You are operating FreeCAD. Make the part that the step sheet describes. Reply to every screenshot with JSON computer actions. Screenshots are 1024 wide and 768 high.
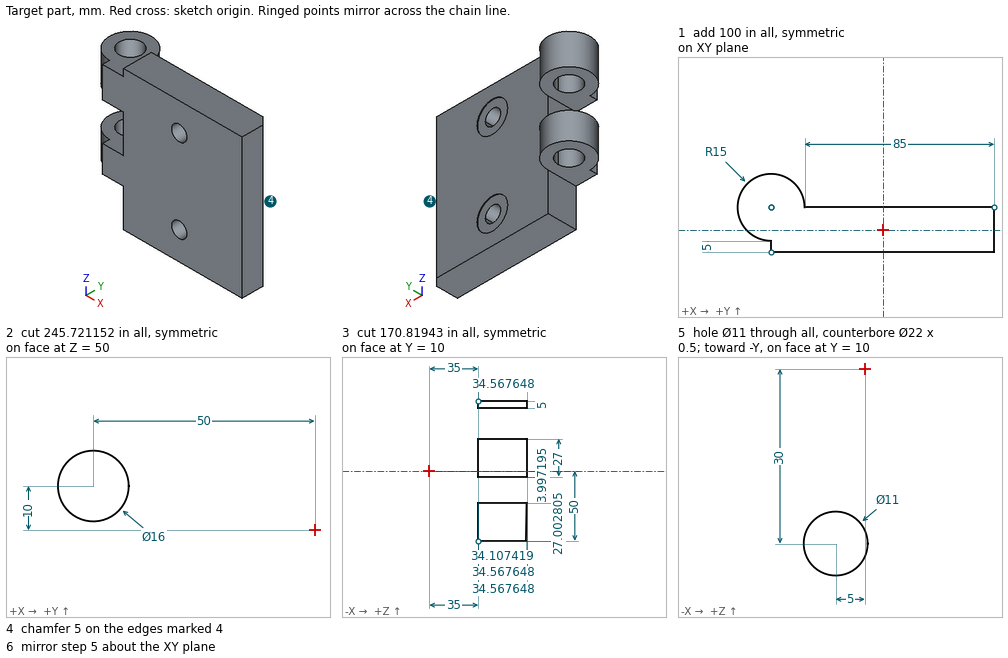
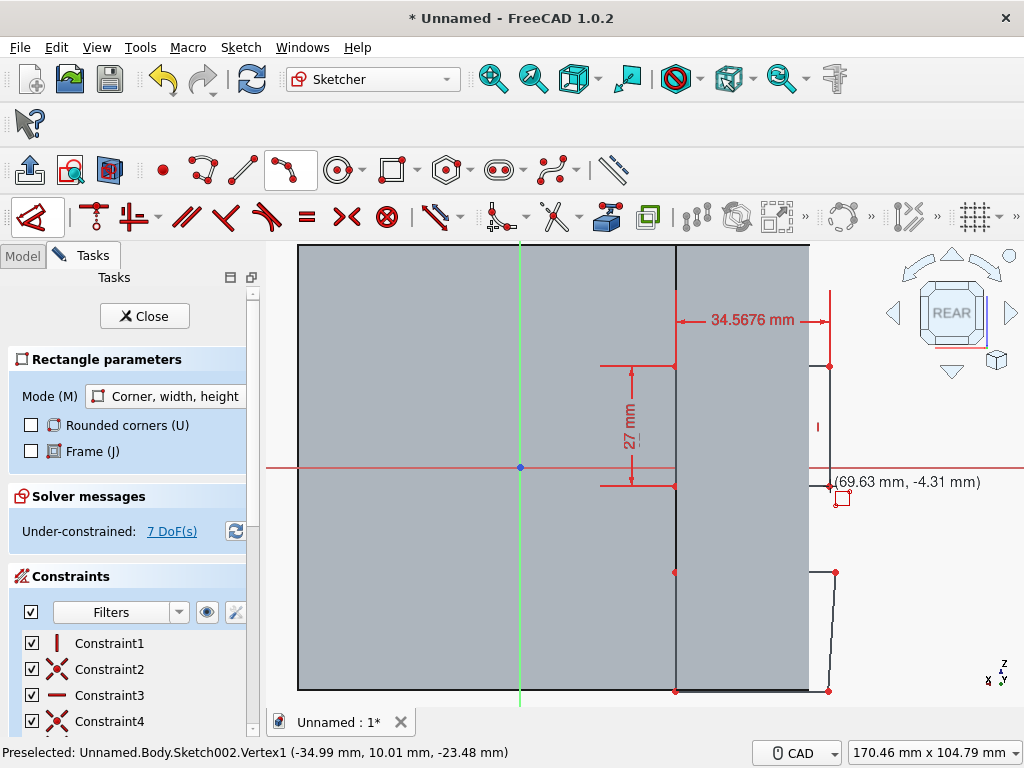
{"action": "scroll", "coordinate": [376, 487], "scroll_direction": "down", "scroll_amount": 2}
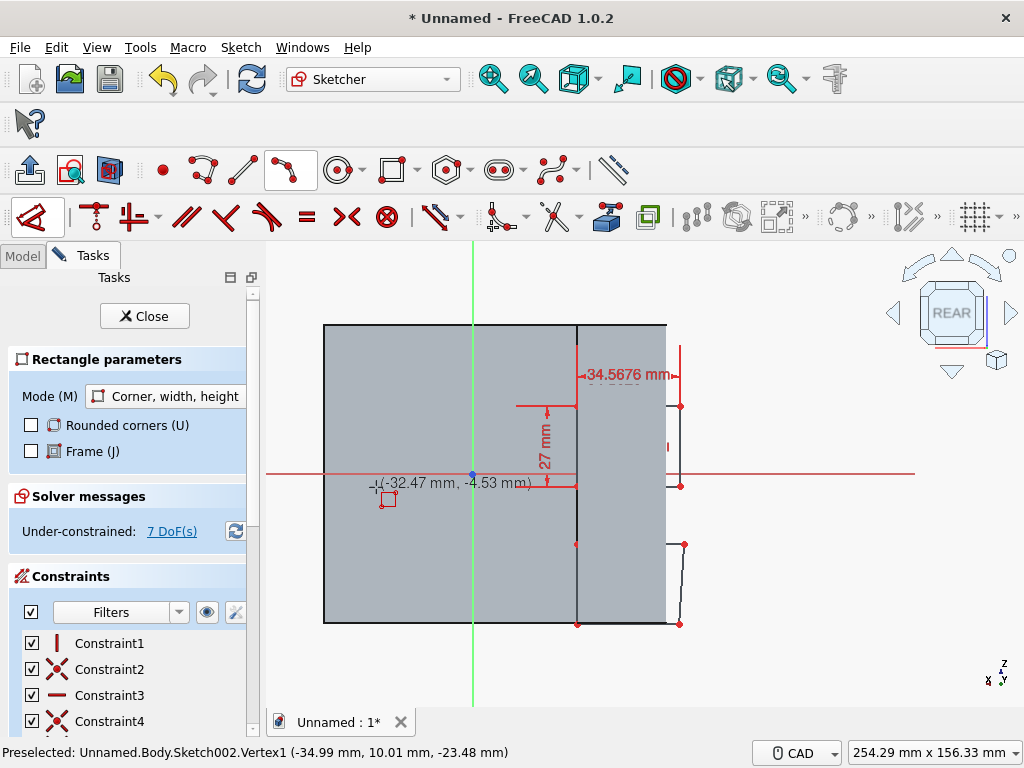
{"action": "left_click", "coordinate": [577, 325]}
{"action": "mouse_move", "coordinate": [680, 340]}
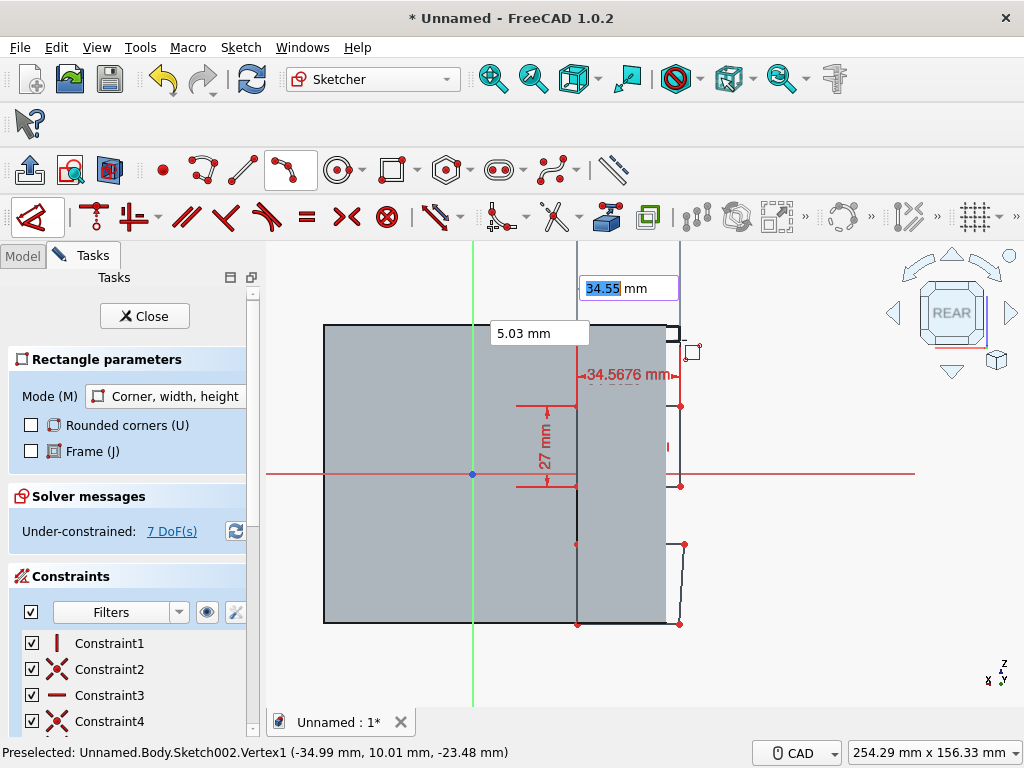
{"action": "type", "text": "34.567648"}
{"action": "key", "text": "Tab"}
{"action": "type", "text": "5"}
{"action": "key", "text": "Return"}
{"action": "key", "text": "Escape"}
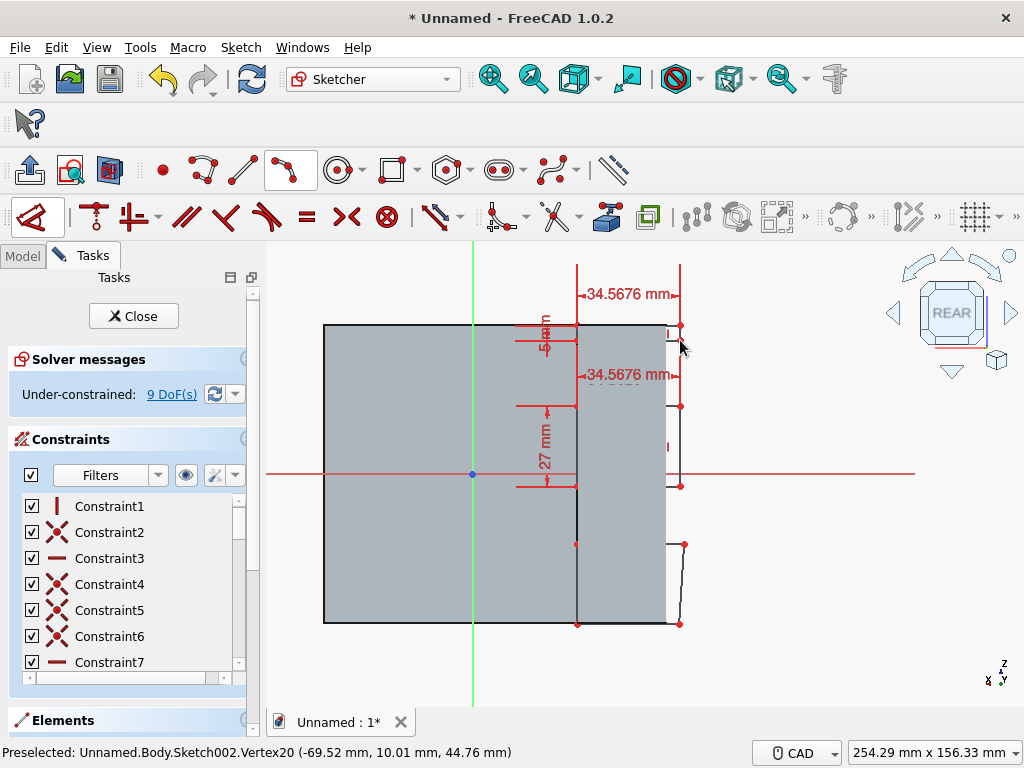
{"action": "left_click", "coordinate": [577, 624]}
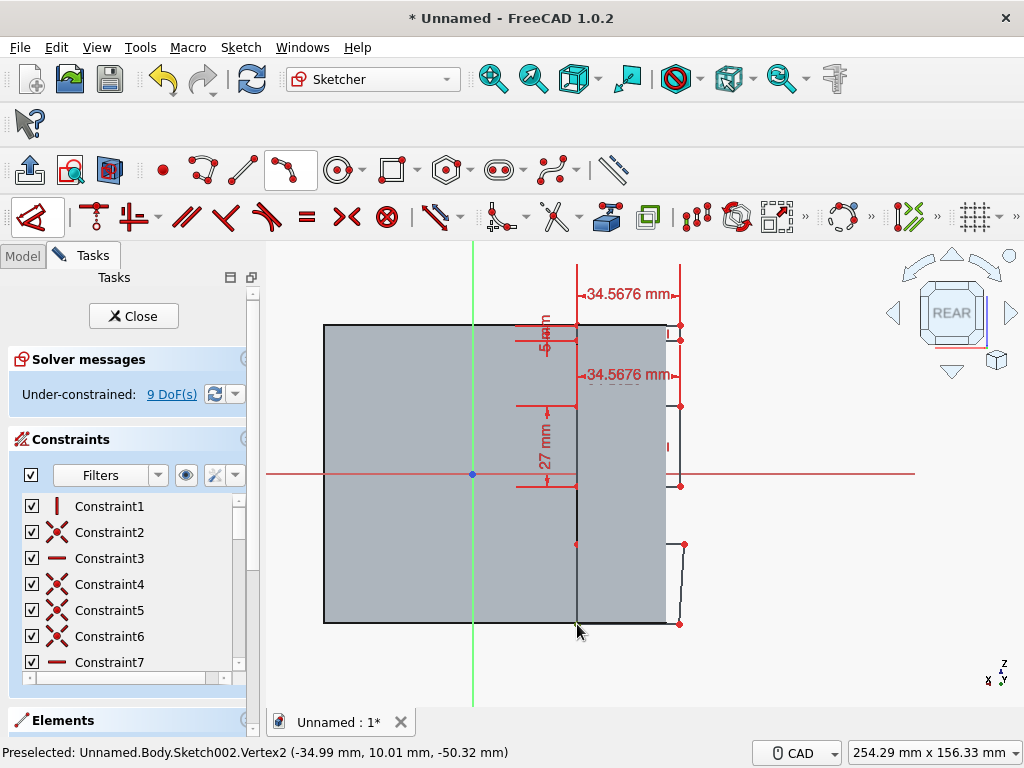
{"action": "left_click", "coordinate": [577, 326]}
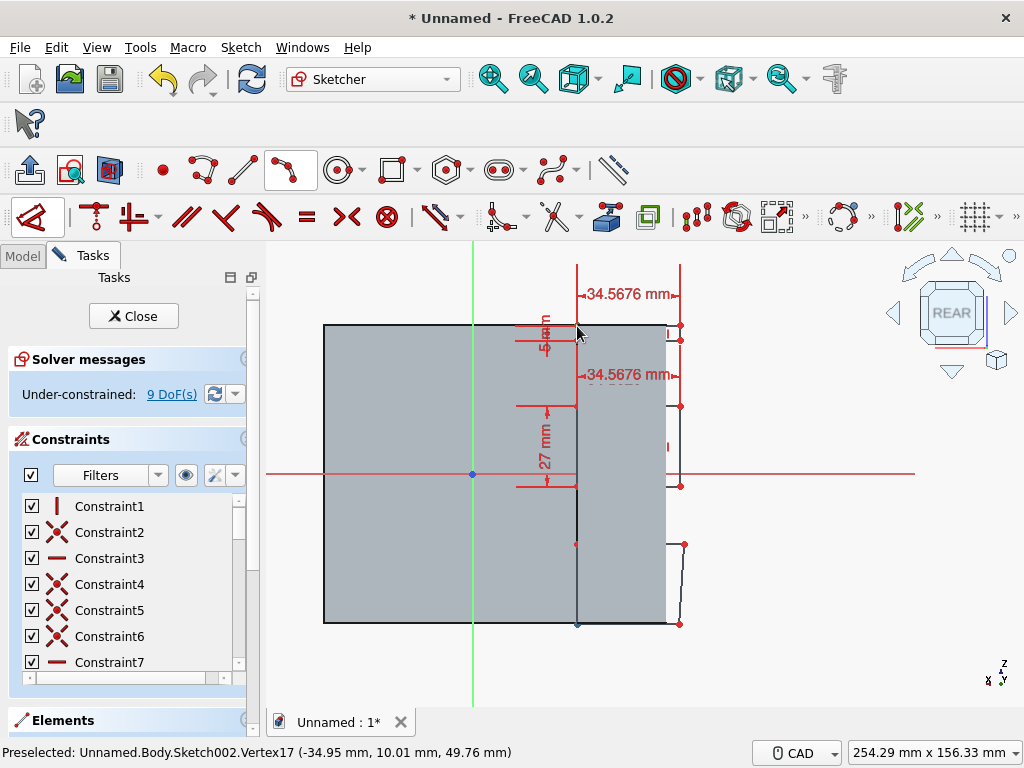
{"action": "left_click", "coordinate": [334, 474]}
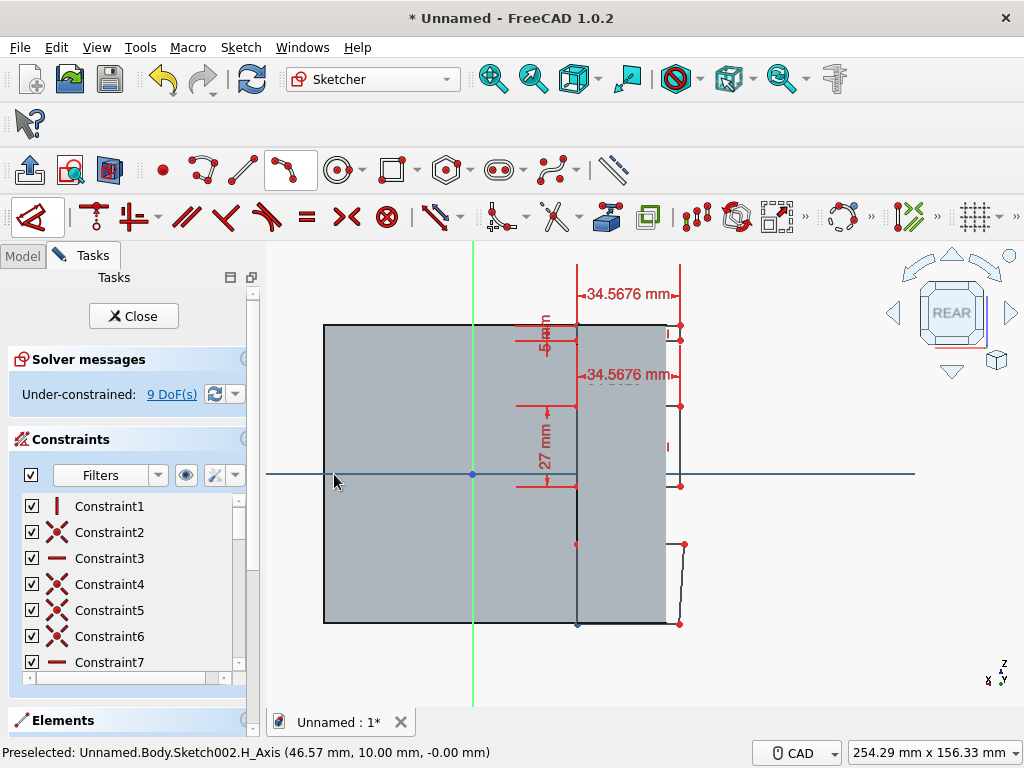
{"action": "left_click", "coordinate": [348, 218]}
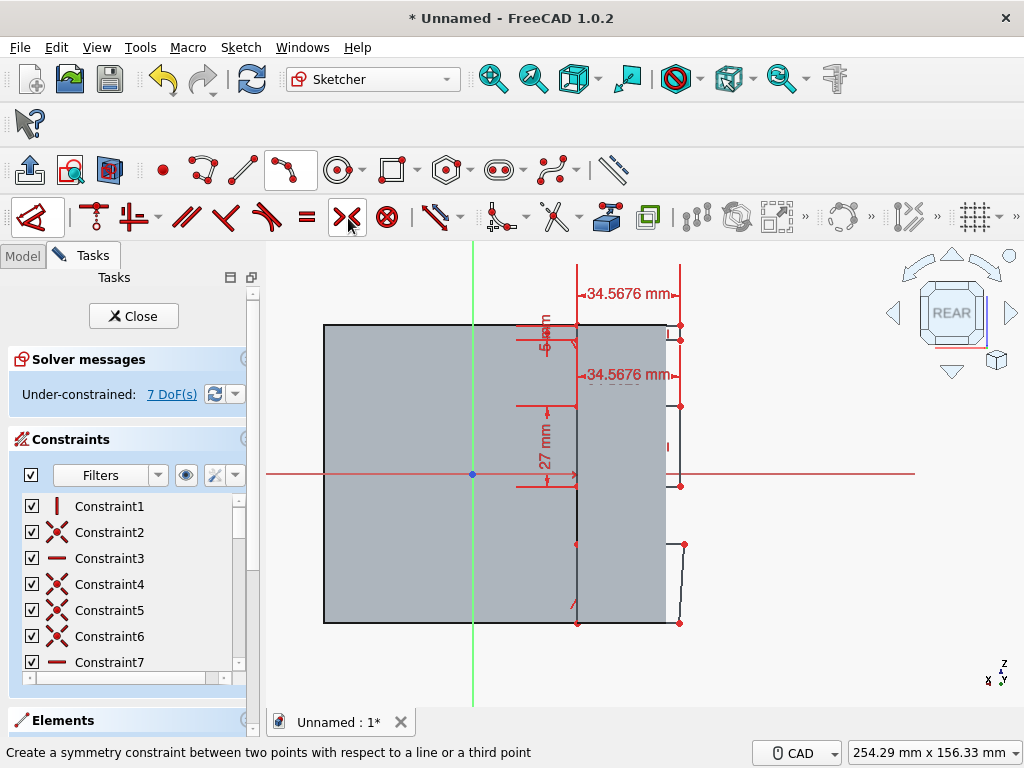
{"action": "left_click", "coordinate": [577, 544]}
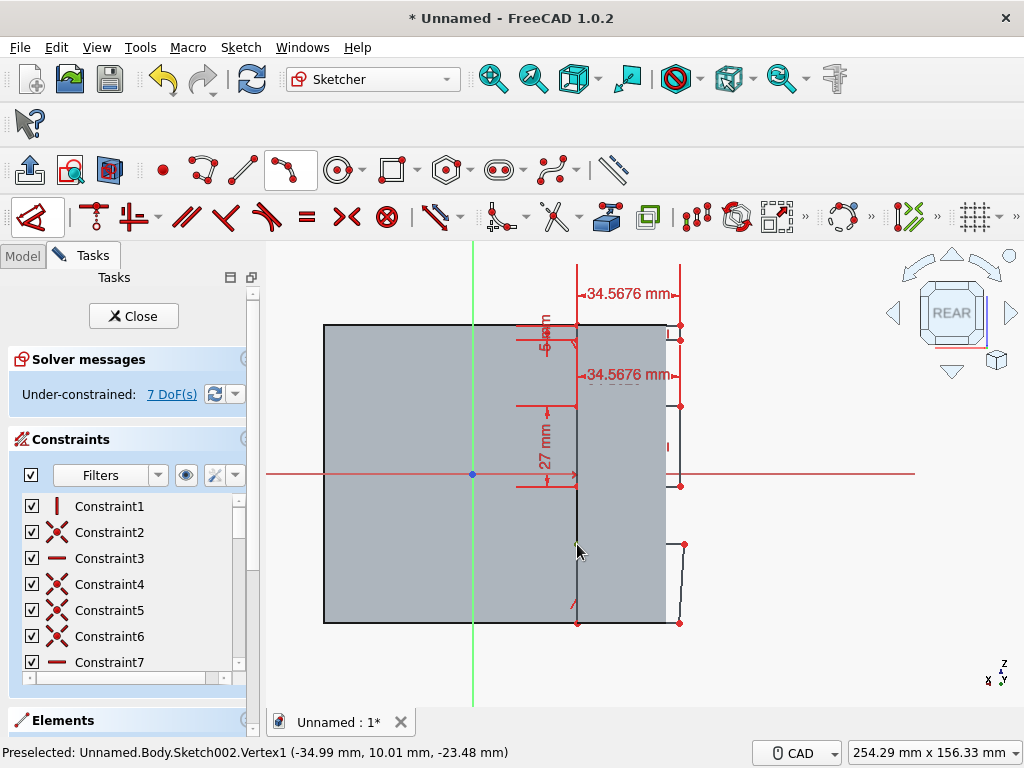
{"action": "left_click", "coordinate": [58, 218]}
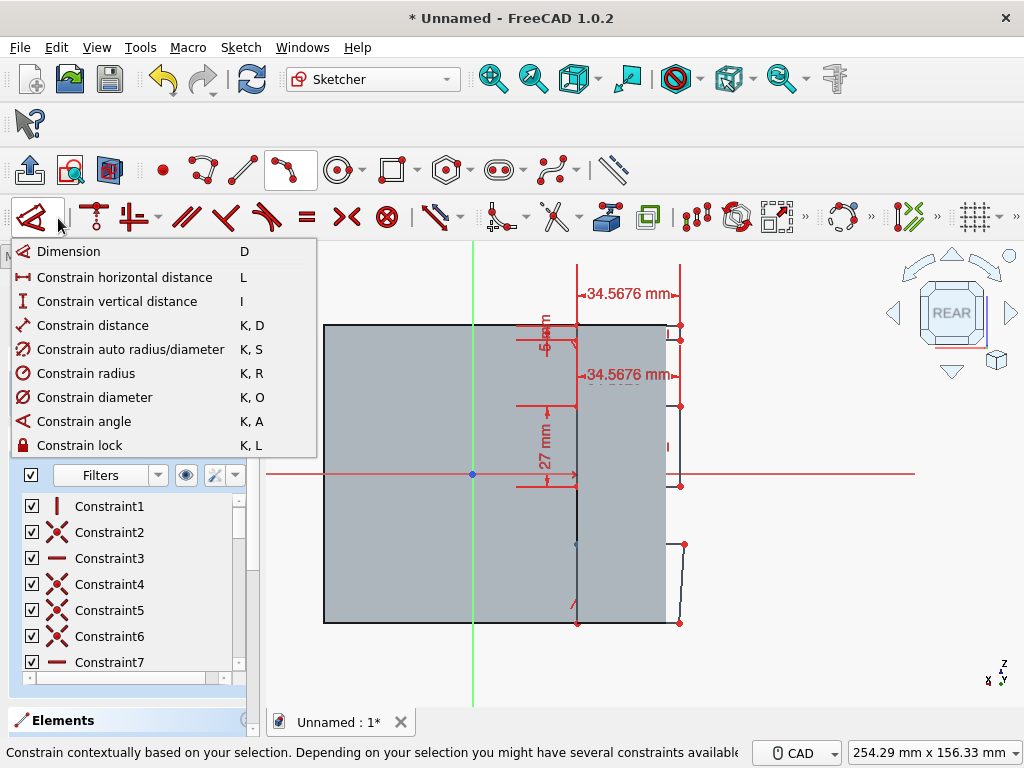
{"action": "left_click", "coordinate": [164, 277]}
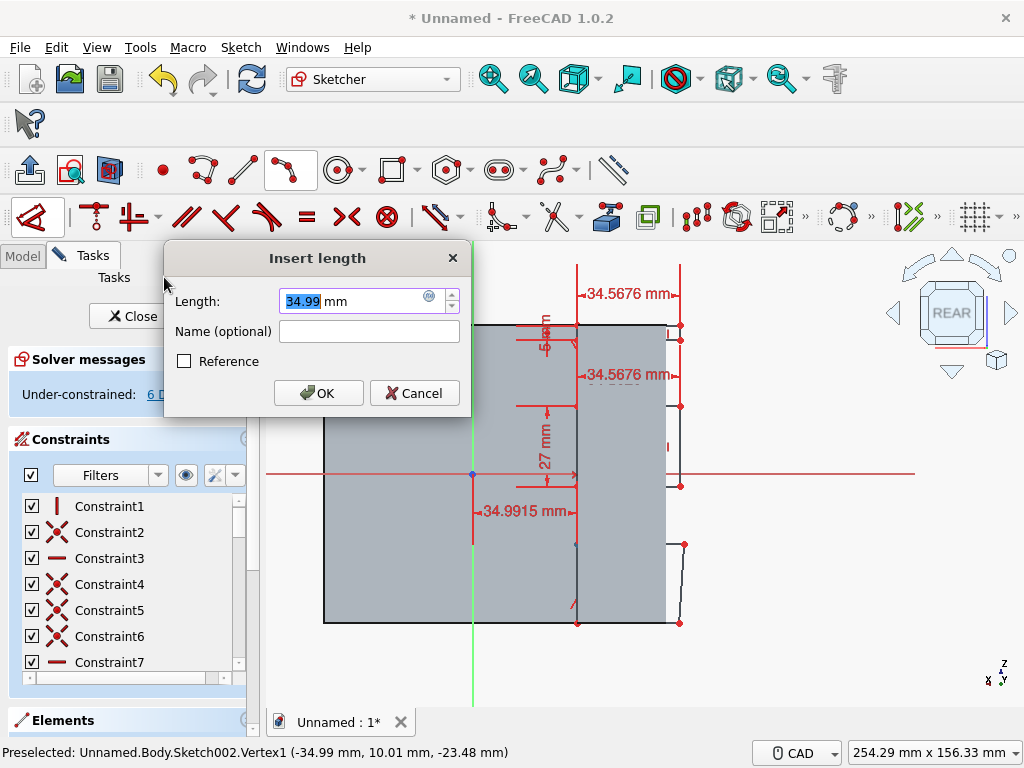
{"action": "type", "text": "35"}
{"action": "key", "text": "Return"}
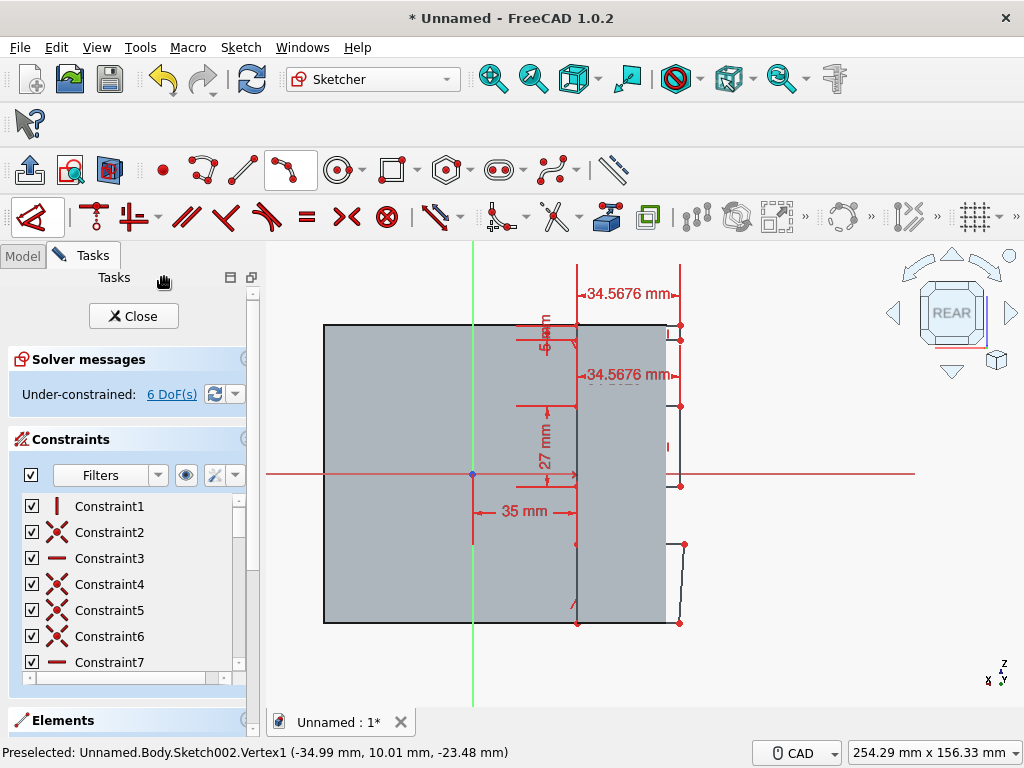
{"action": "left_click", "coordinate": [577, 623]}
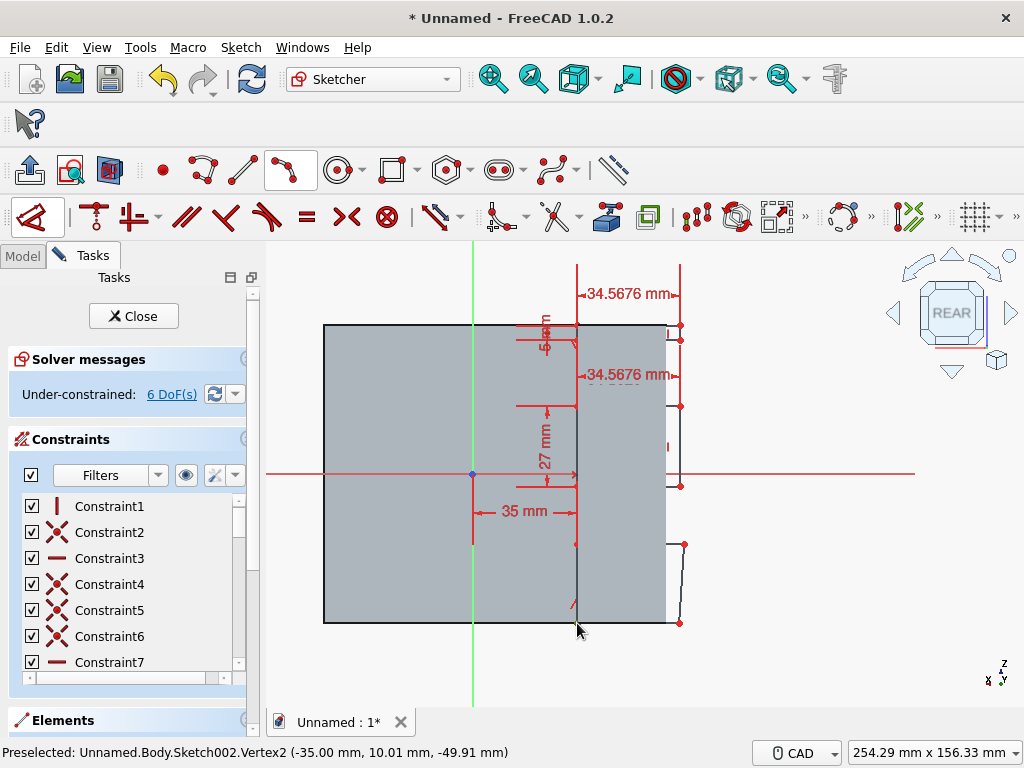
{"action": "left_click", "coordinate": [58, 218]}